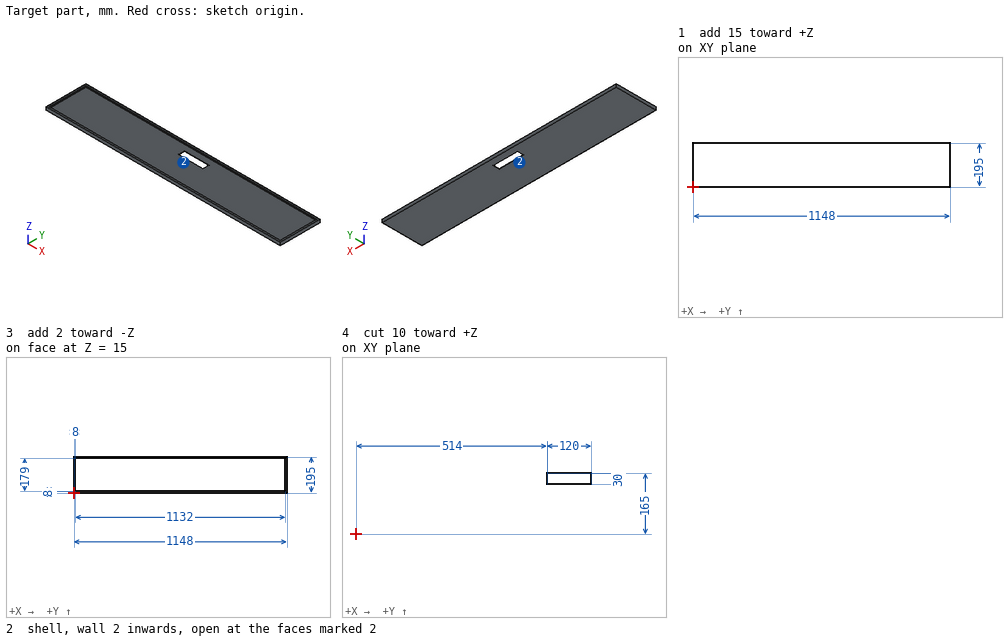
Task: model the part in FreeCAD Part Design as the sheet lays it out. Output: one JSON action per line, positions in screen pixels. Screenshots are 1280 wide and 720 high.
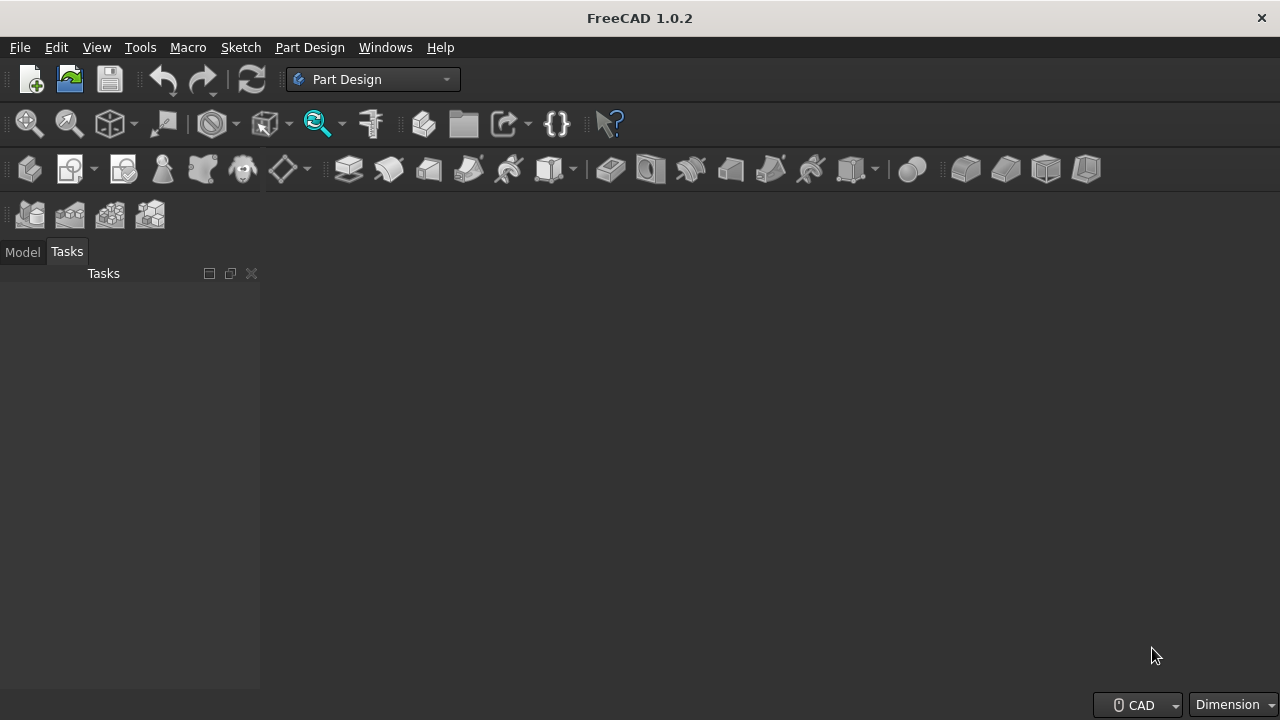
{"action": "left_click", "coordinate": [30, 80]}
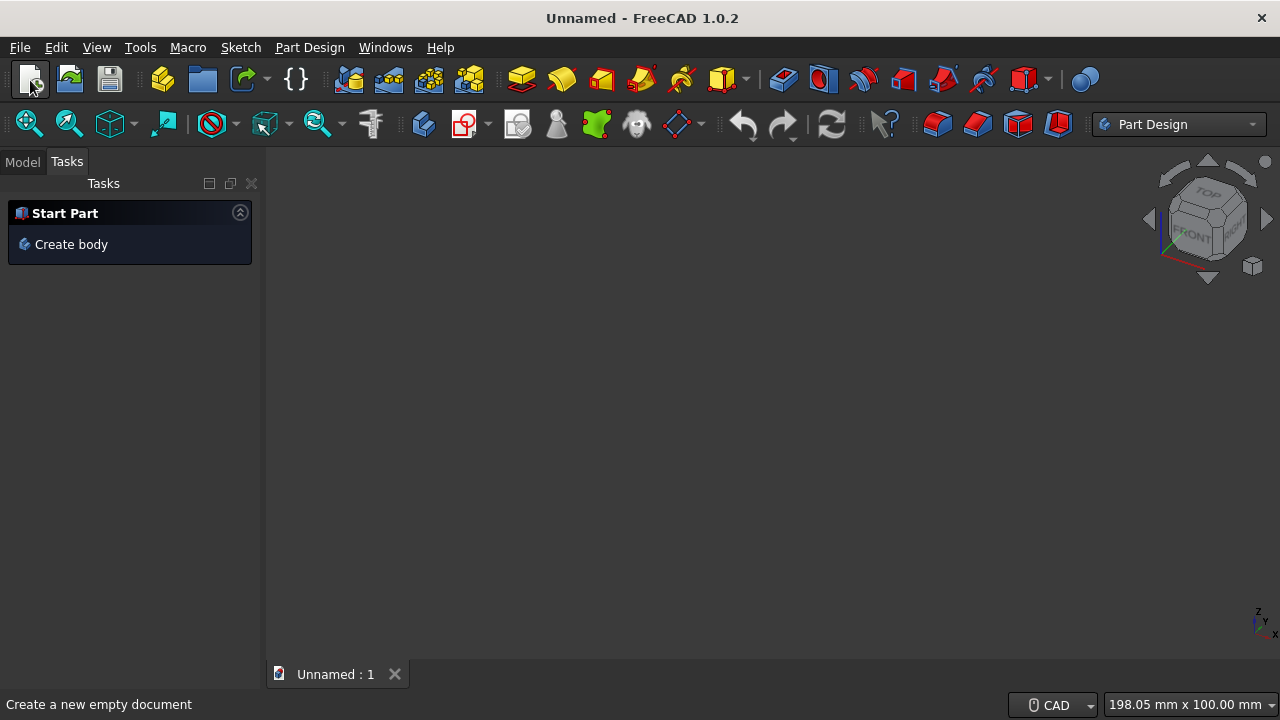
{"action": "left_click", "coordinate": [464, 124]}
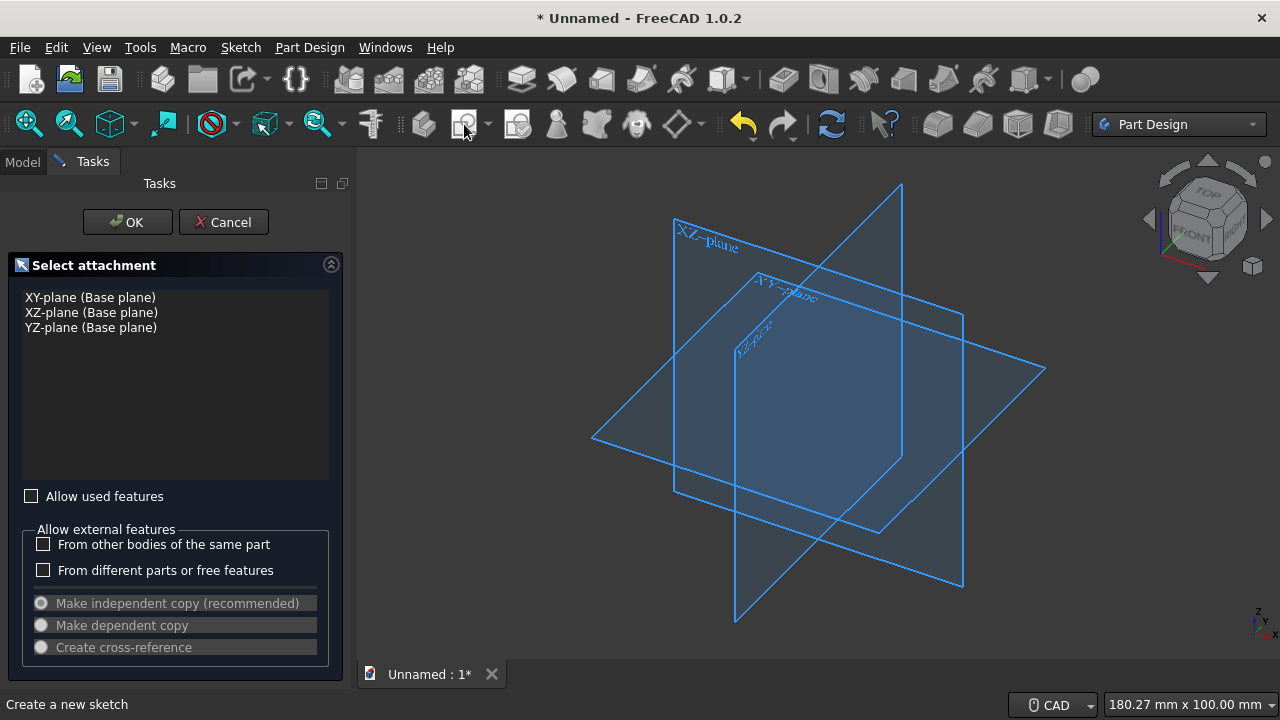
{"action": "left_click", "coordinate": [82, 298]}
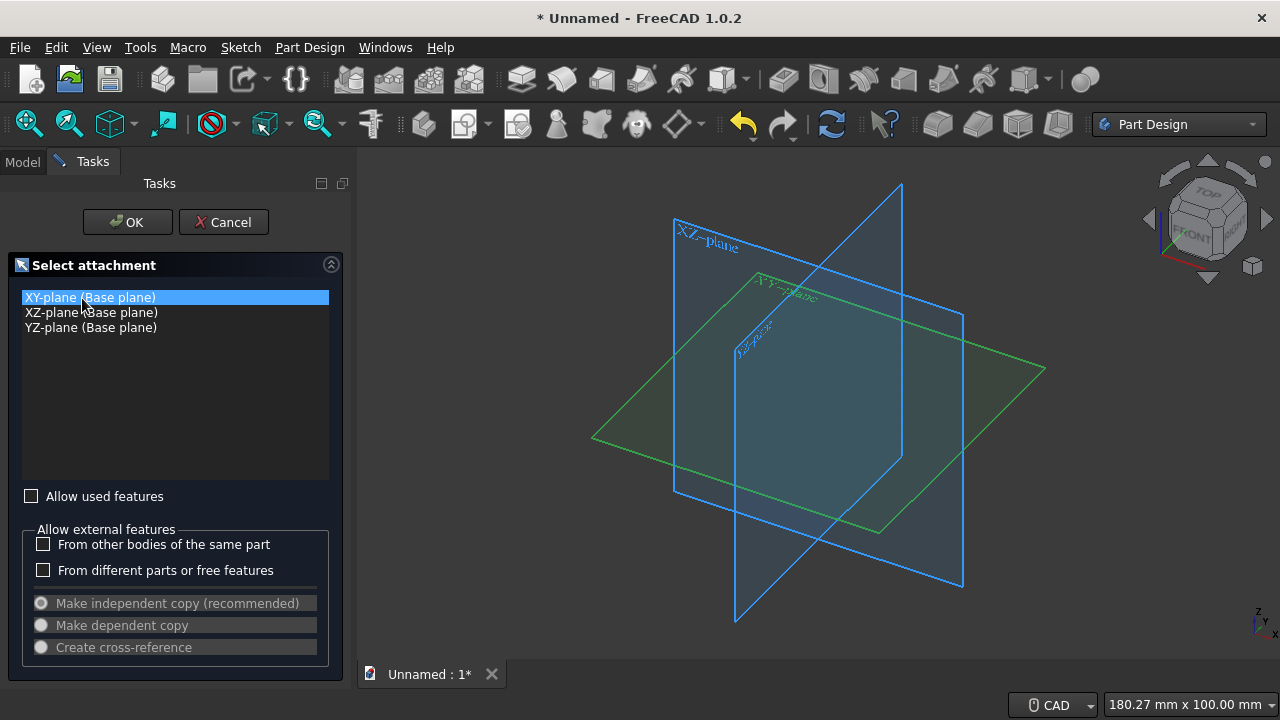
{"action": "left_click", "coordinate": [128, 222]}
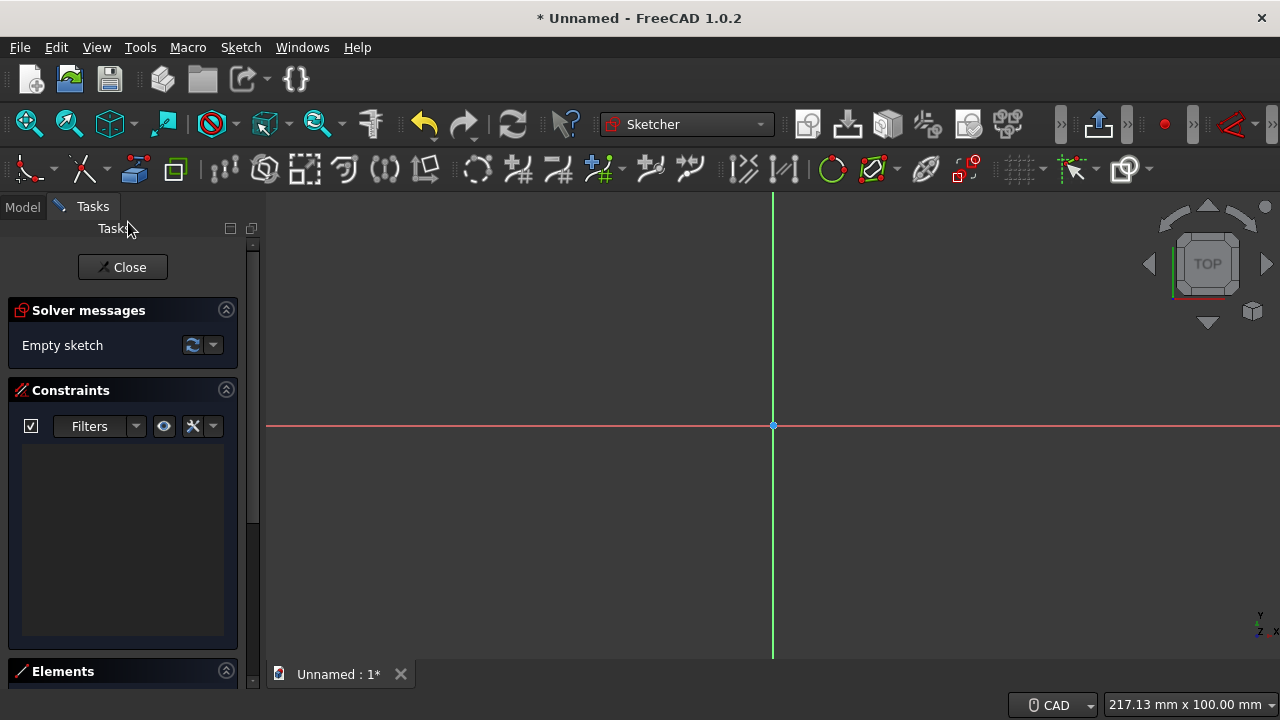
{"action": "scroll", "coordinate": [362, 482], "scroll_direction": "down", "scroll_amount": 11}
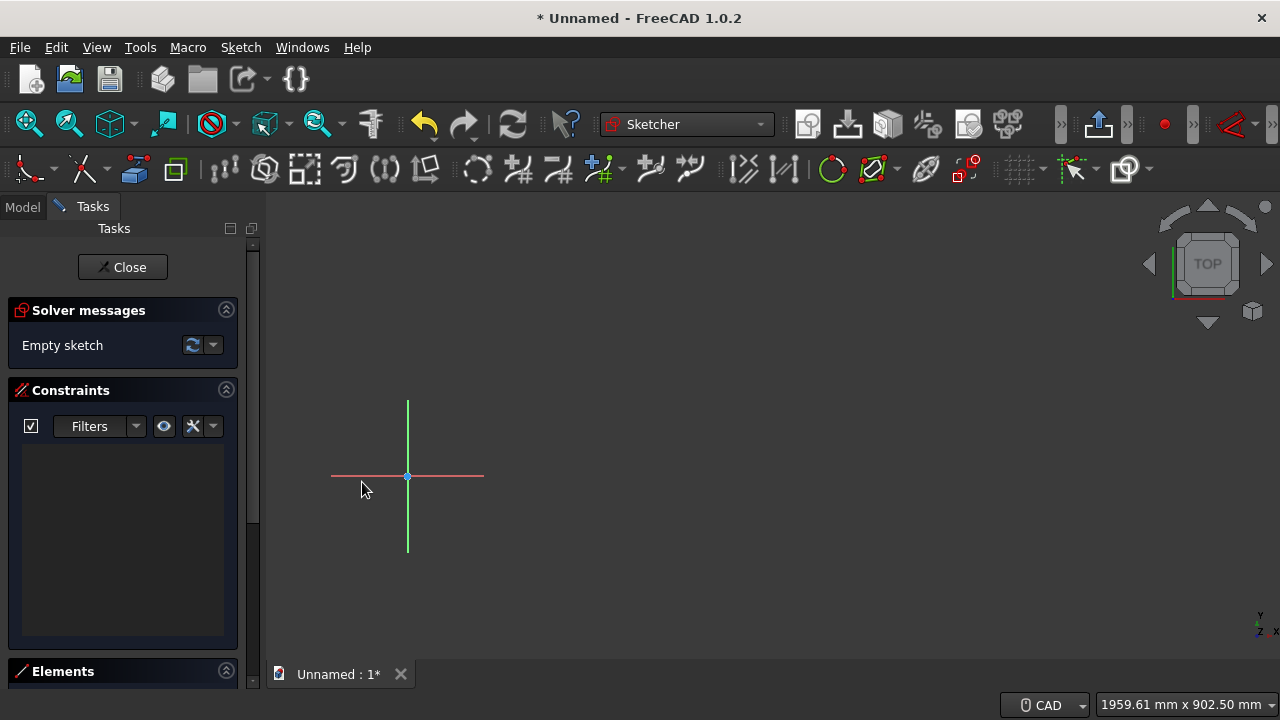
{"action": "key", "text": "g r"}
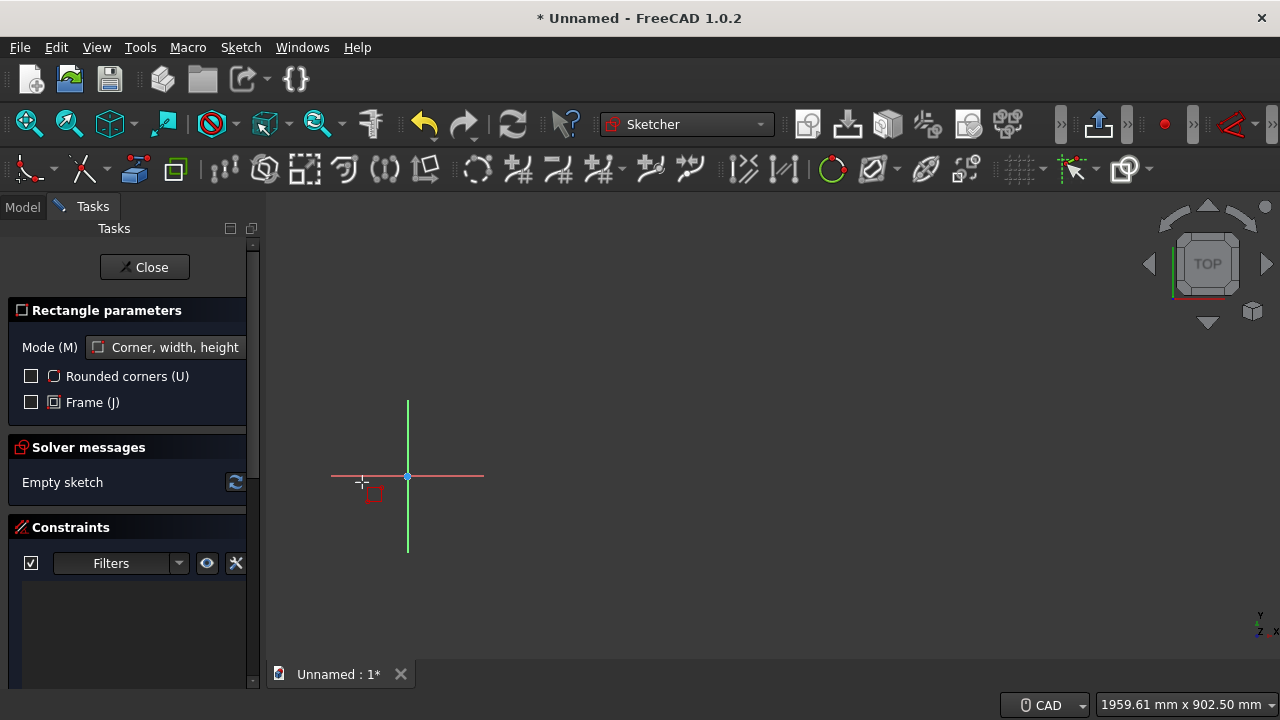
{"action": "left_click", "coordinate": [408, 476]}
{"action": "mouse_move", "coordinate": [1002, 375]}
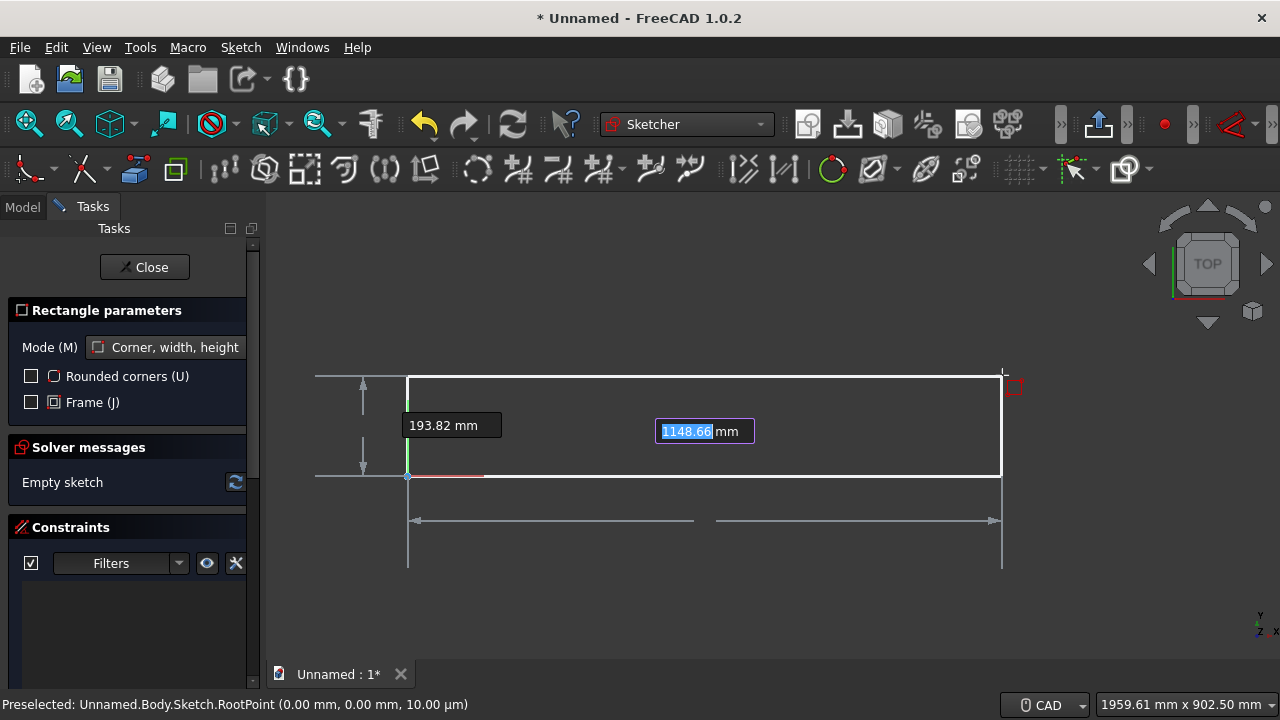
{"action": "type", "text": "1148"}
{"action": "key", "text": "Tab"}
{"action": "type", "text": "195"}
{"action": "key", "text": "Return"}
{"action": "key", "text": "Escape"}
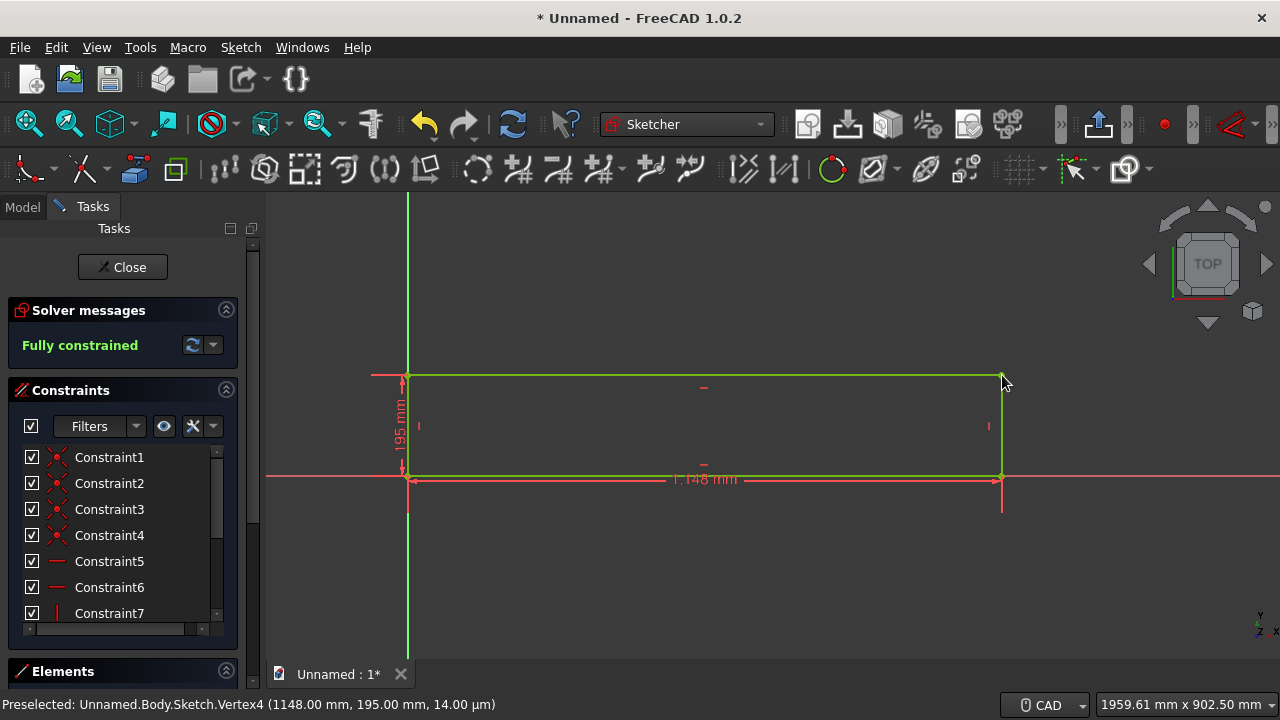
{"action": "left_click", "coordinate": [123, 267]}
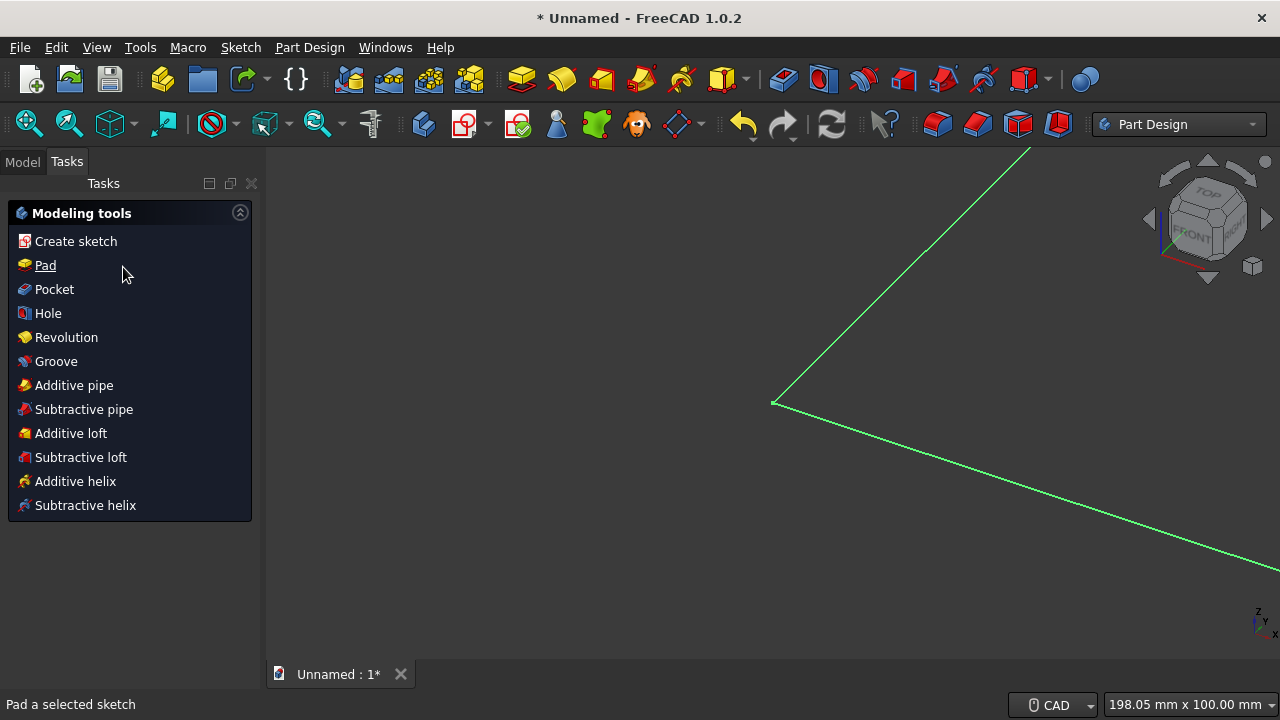
{"action": "left_click", "coordinate": [522, 80]}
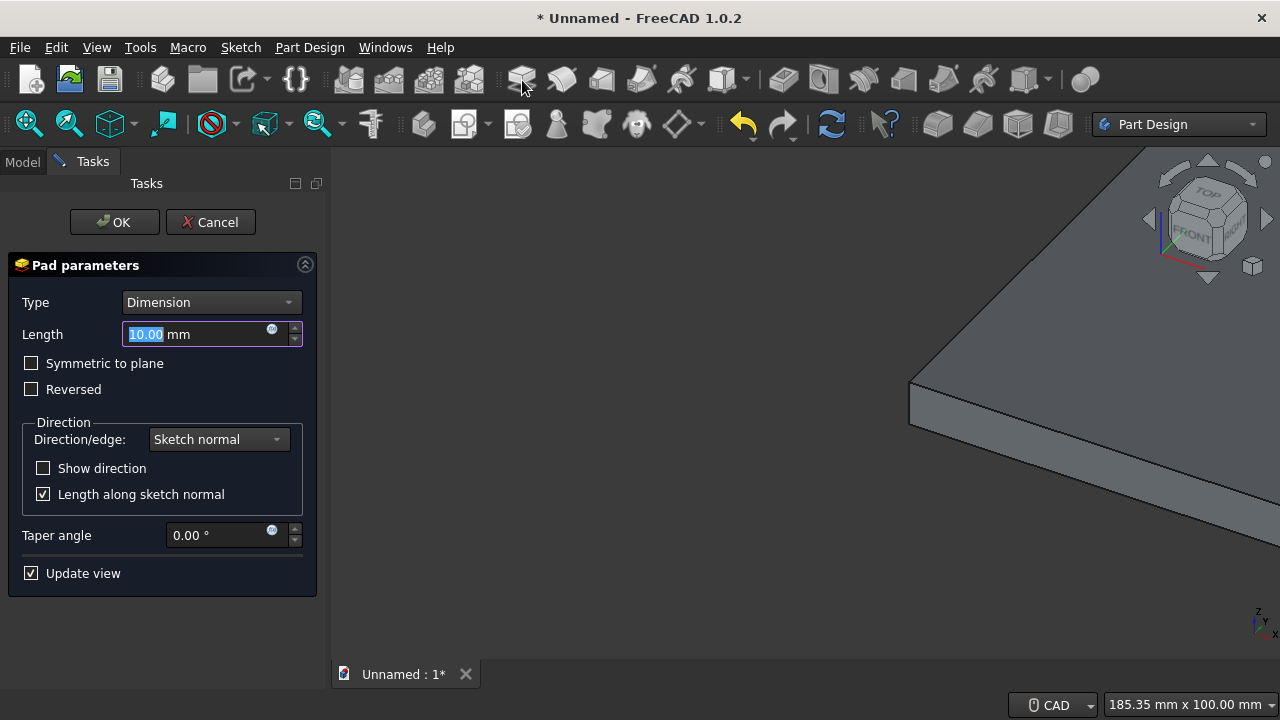
{"action": "type", "text": "15"}
{"action": "key", "text": "Tab"}